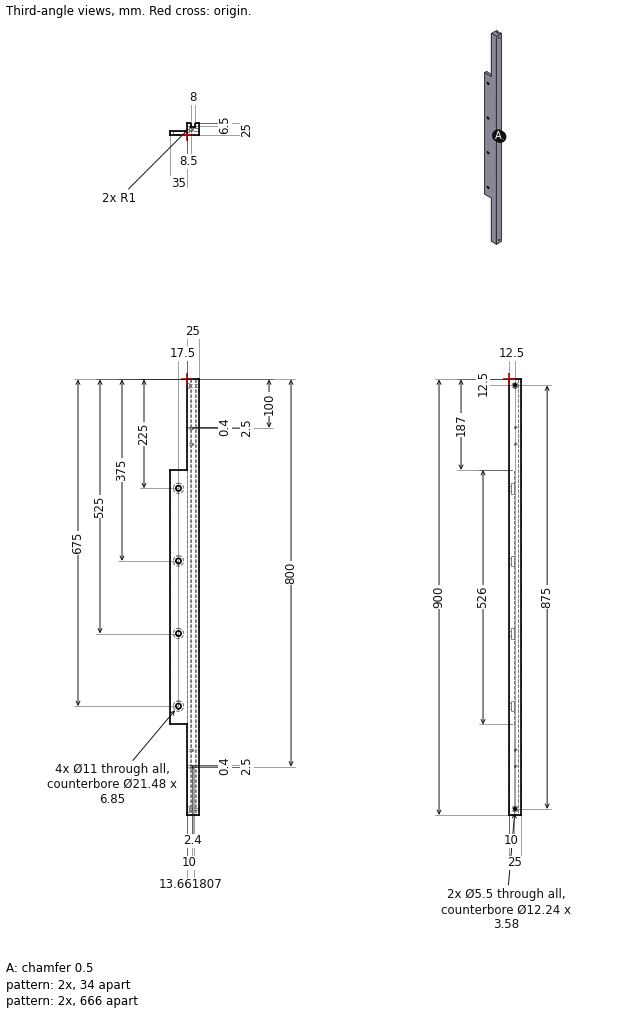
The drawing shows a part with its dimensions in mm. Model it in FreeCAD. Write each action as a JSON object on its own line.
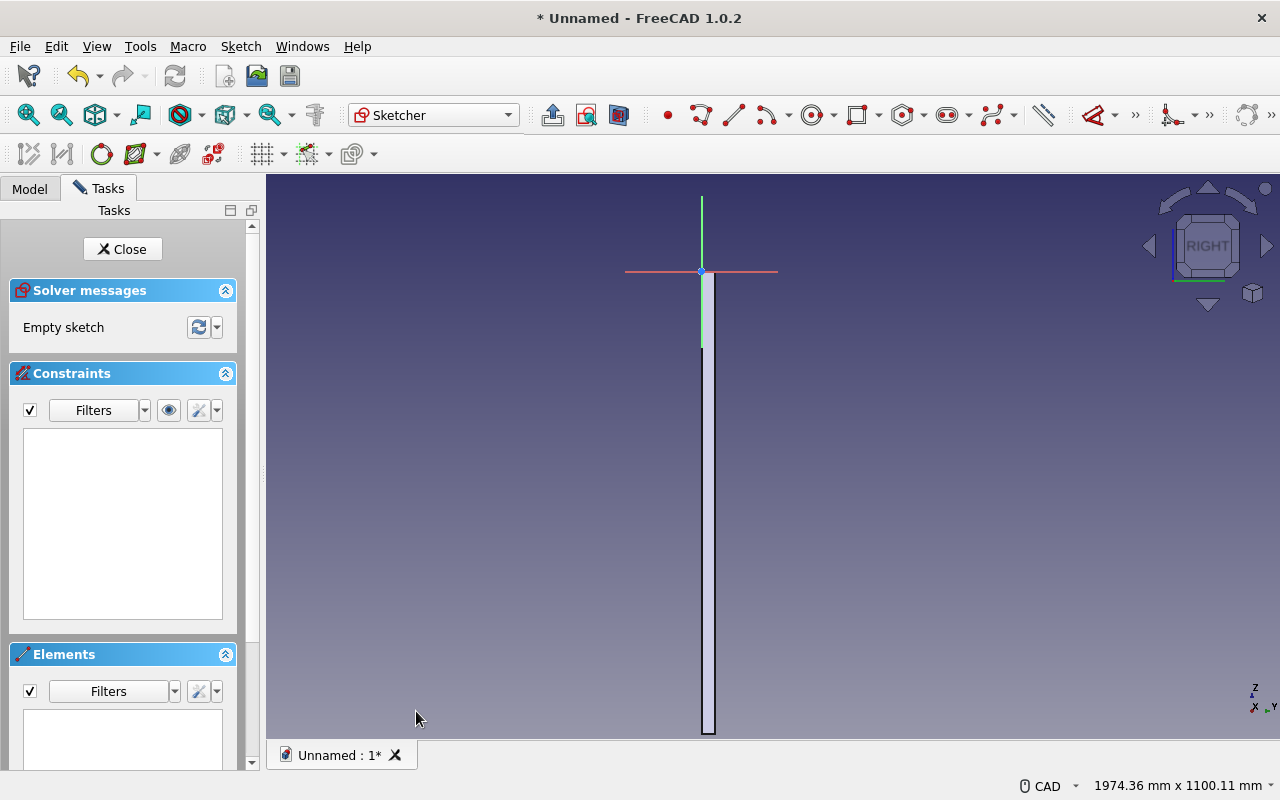
{"action": "left_click", "coordinate": [856, 116]}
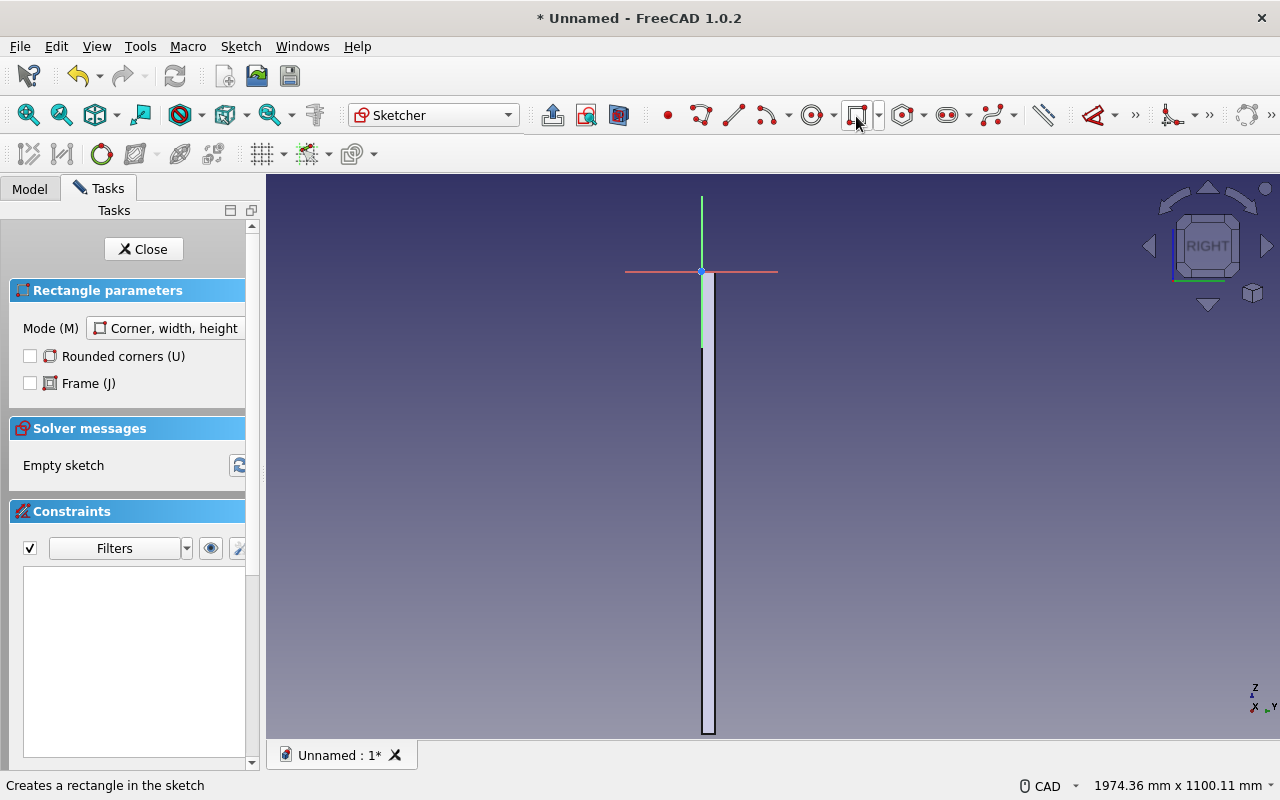
{"action": "scroll", "coordinate": [702, 368], "scroll_direction": "up", "scroll_amount": 6}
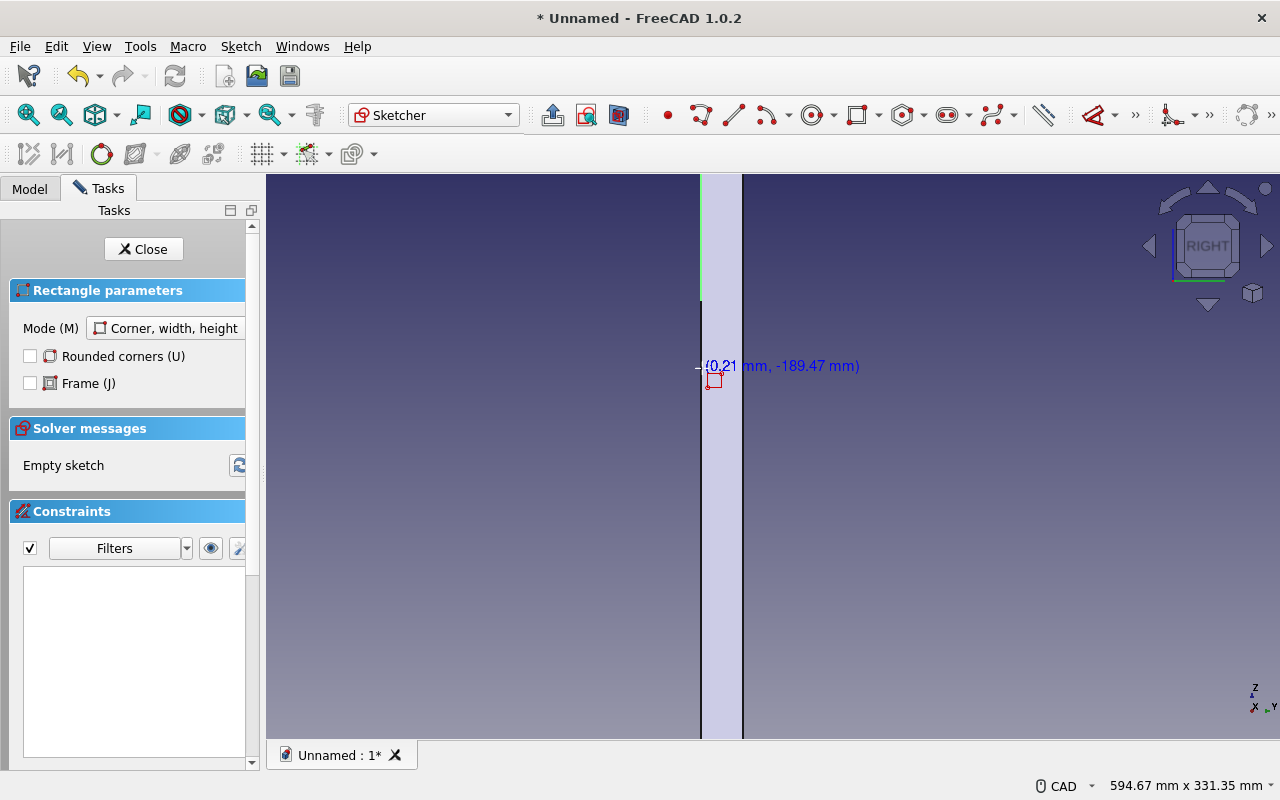
{"action": "left_click", "coordinate": [701, 366]}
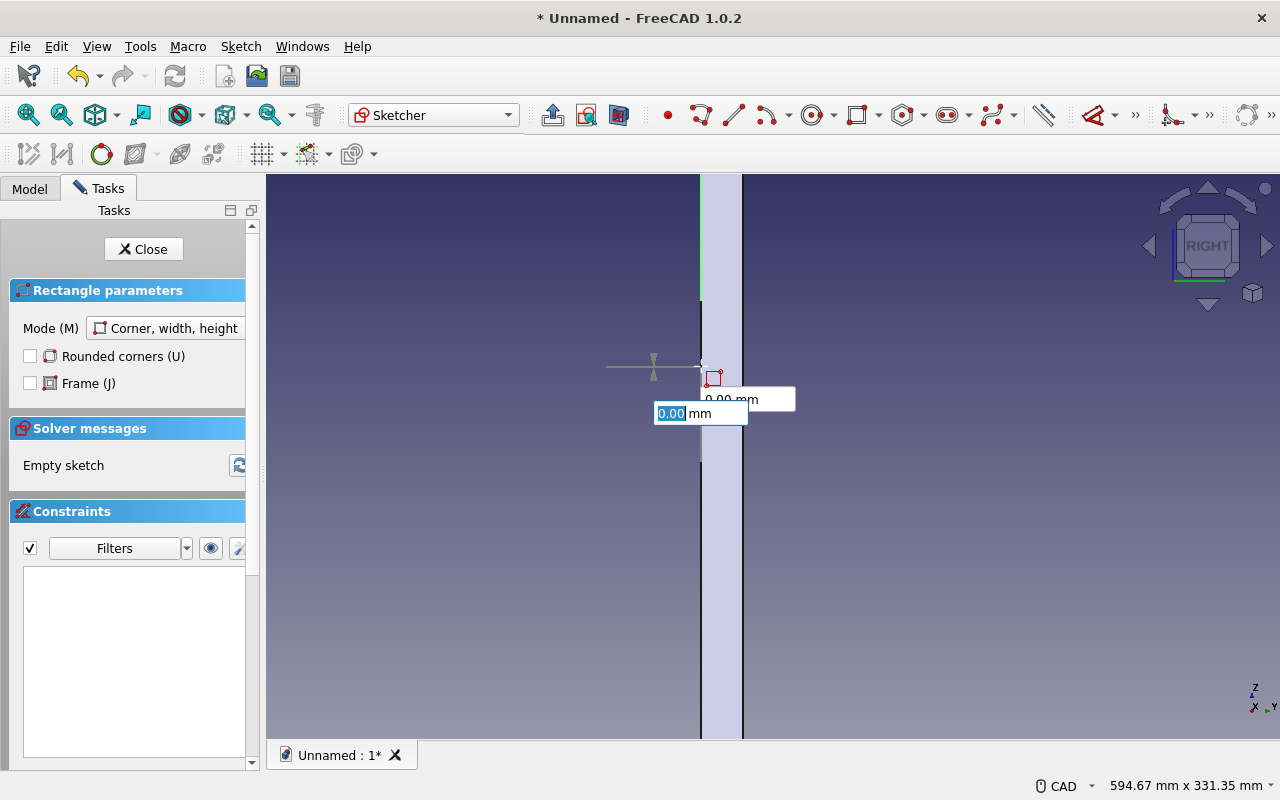
{"action": "scroll", "coordinate": [702, 371], "scroll_direction": "down", "scroll_amount": 6}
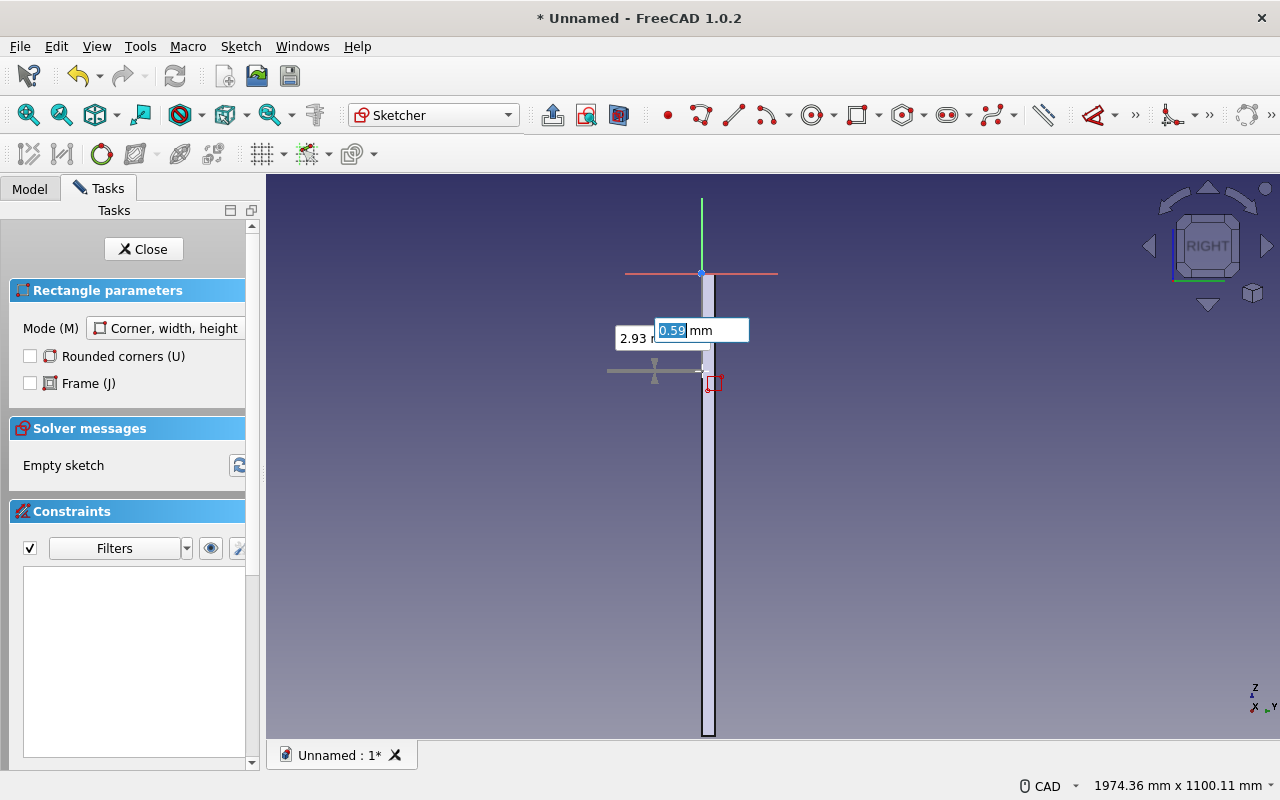
{"action": "scroll", "coordinate": [707, 640], "scroll_direction": "up", "scroll_amount": 6}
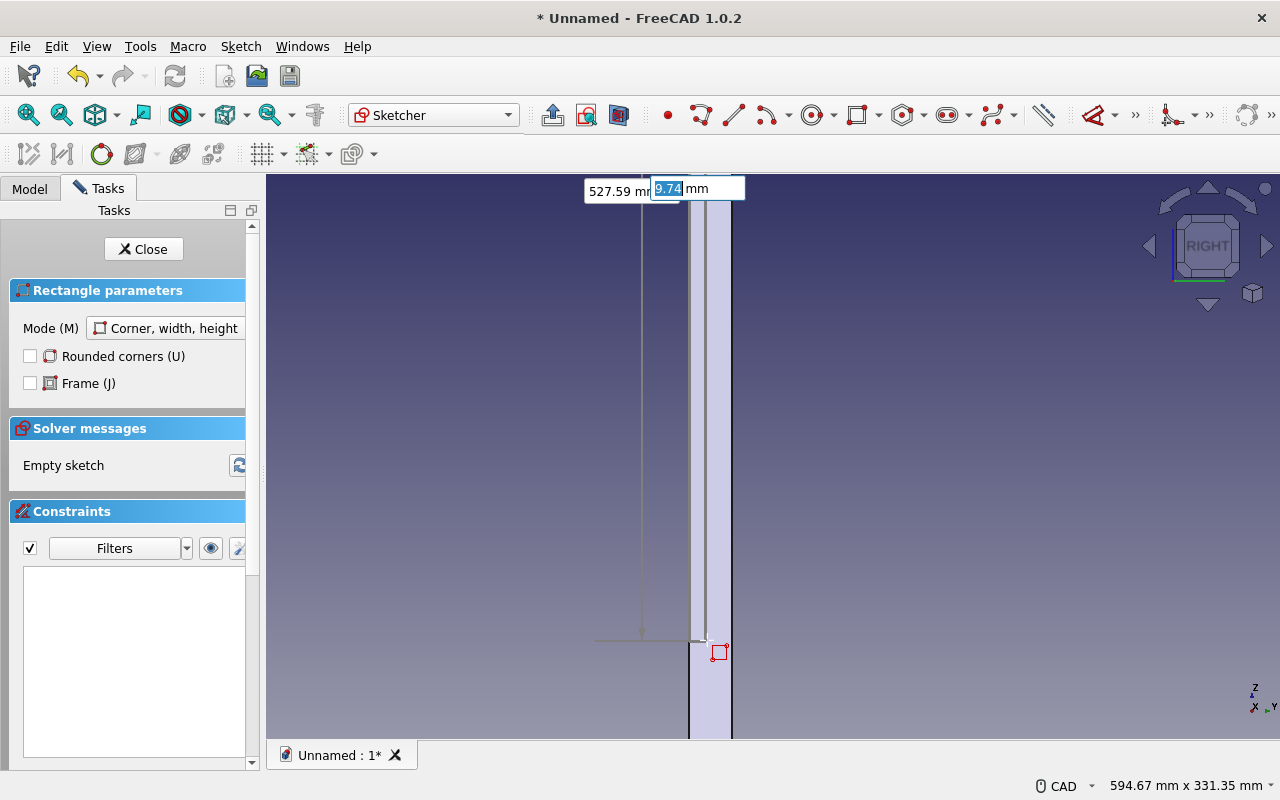
{"action": "left_click", "coordinate": [706, 638]}
{"action": "key", "text": "Escape"}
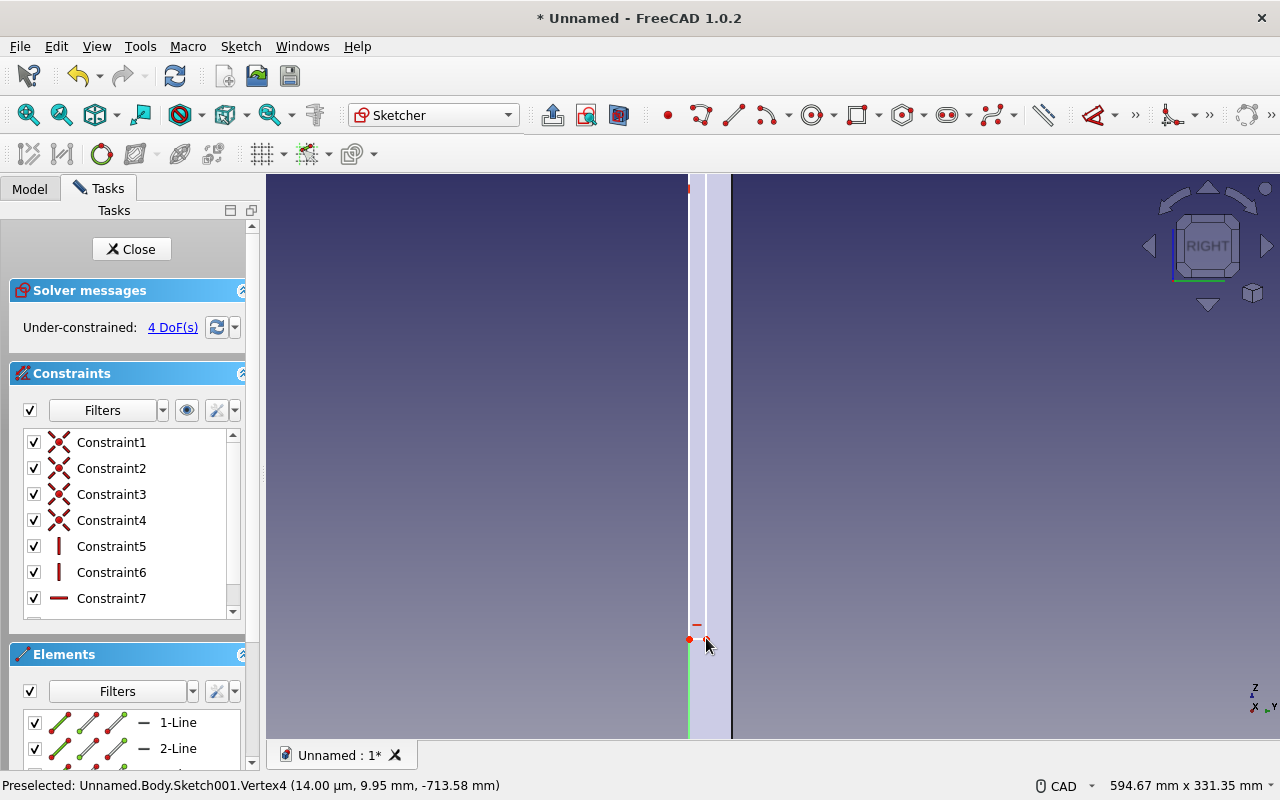
{"action": "scroll", "coordinate": [707, 640], "scroll_direction": "down", "scroll_amount": 6}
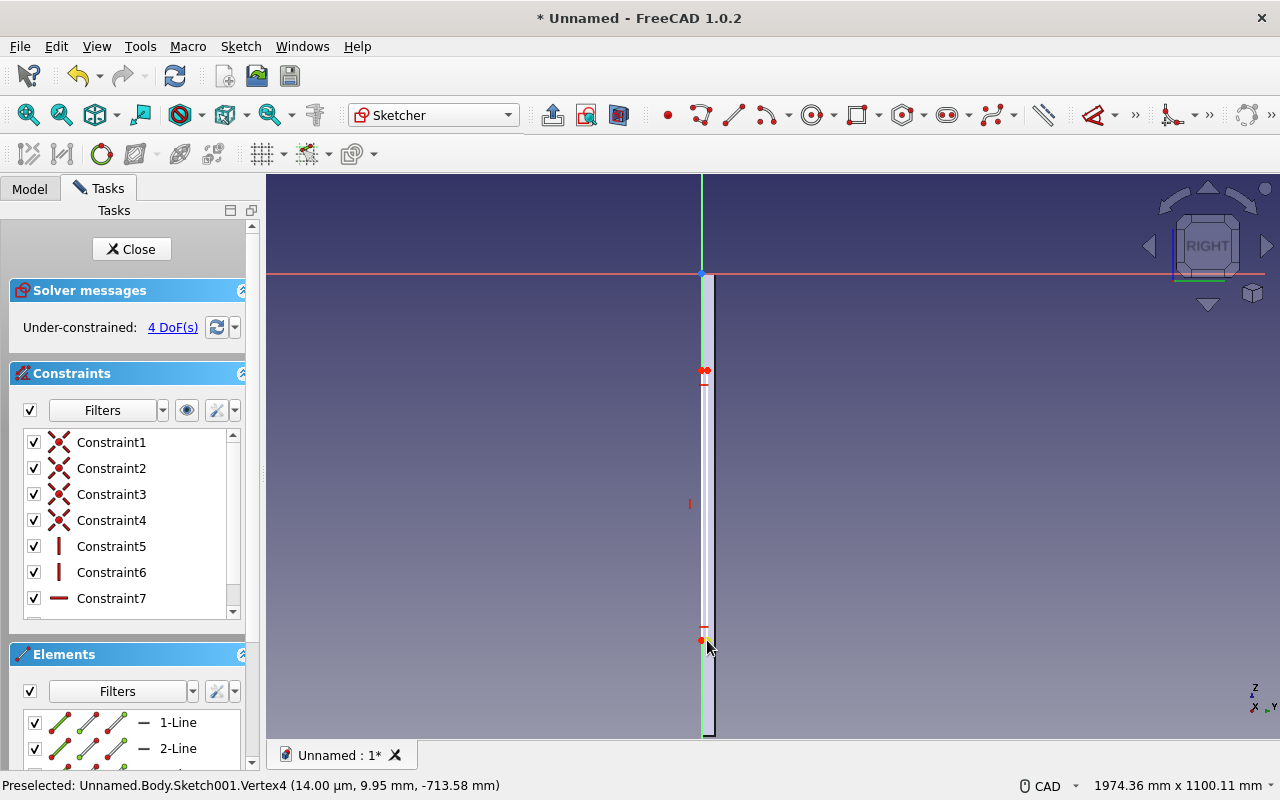
{"action": "scroll", "coordinate": [702, 370], "scroll_direction": "up", "scroll_amount": 5}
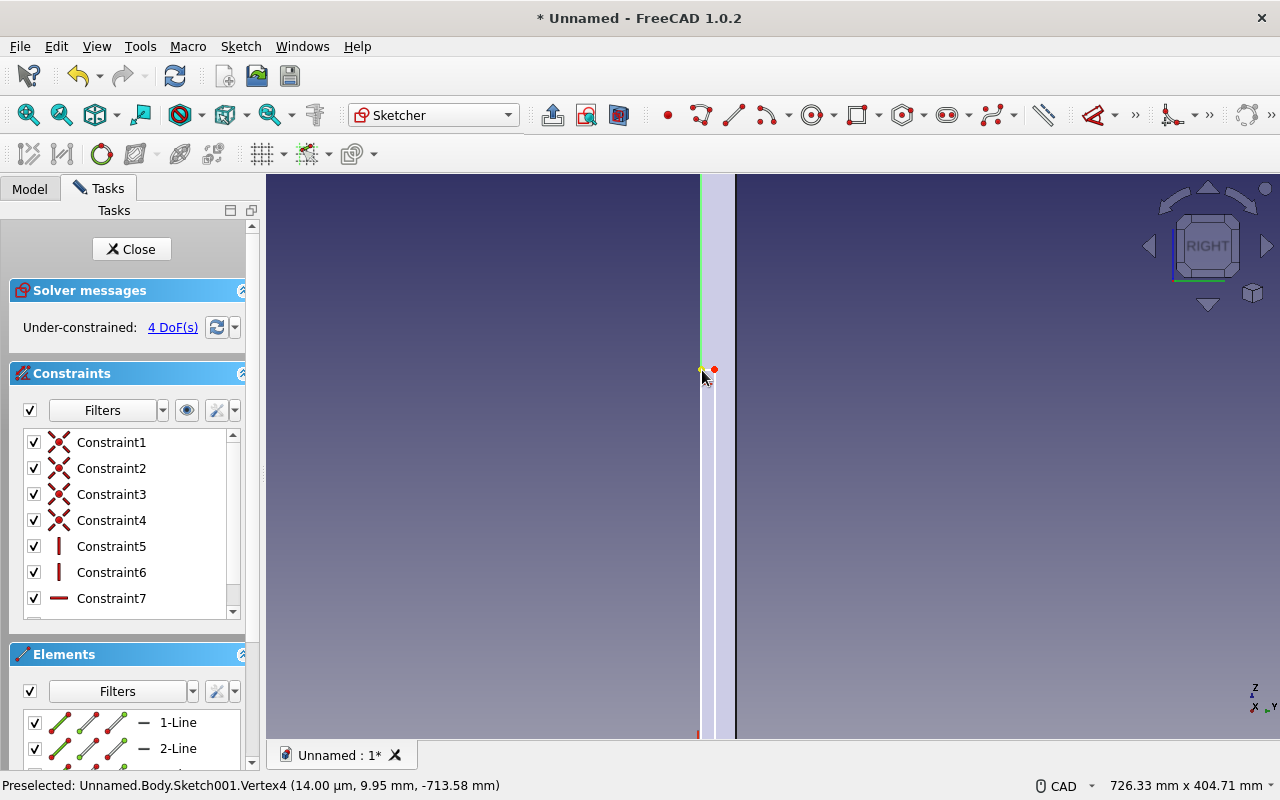
{"action": "left_click", "coordinate": [701, 370]}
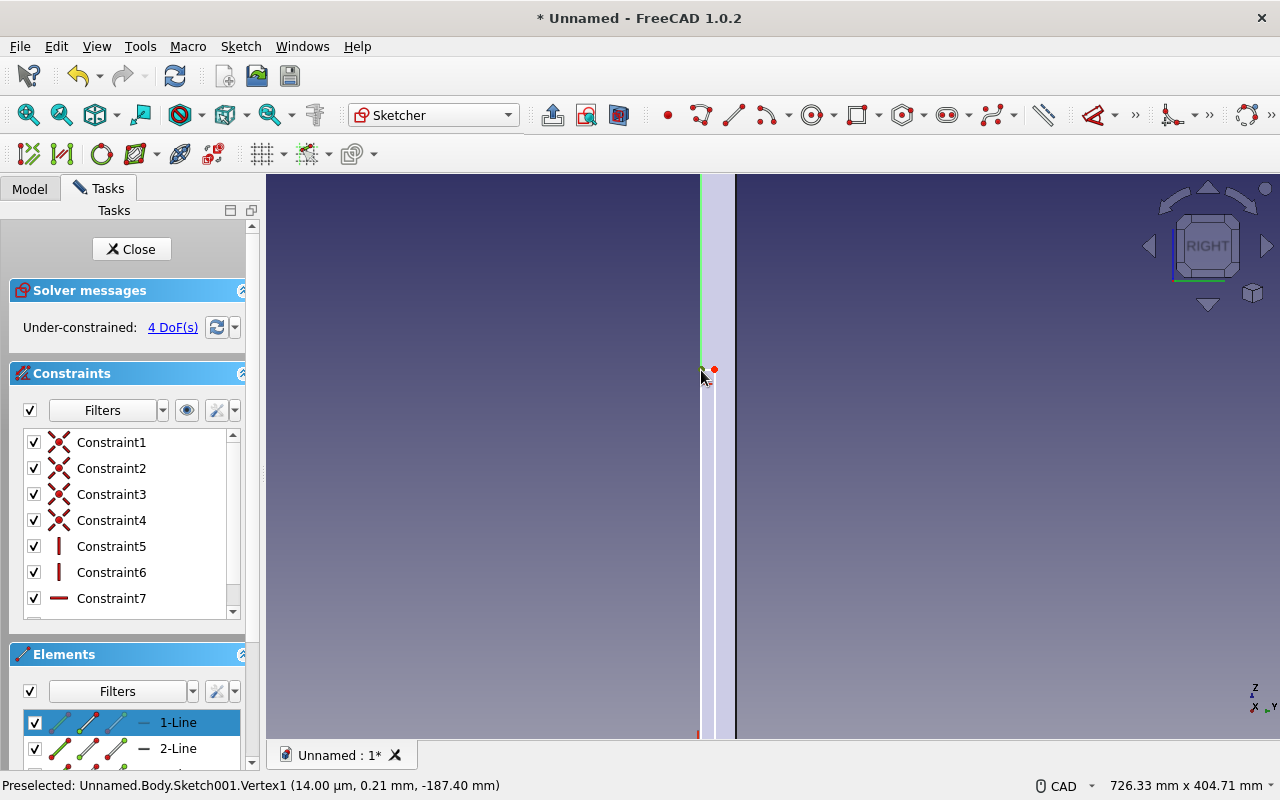
{"action": "left_click", "coordinate": [701, 311]}